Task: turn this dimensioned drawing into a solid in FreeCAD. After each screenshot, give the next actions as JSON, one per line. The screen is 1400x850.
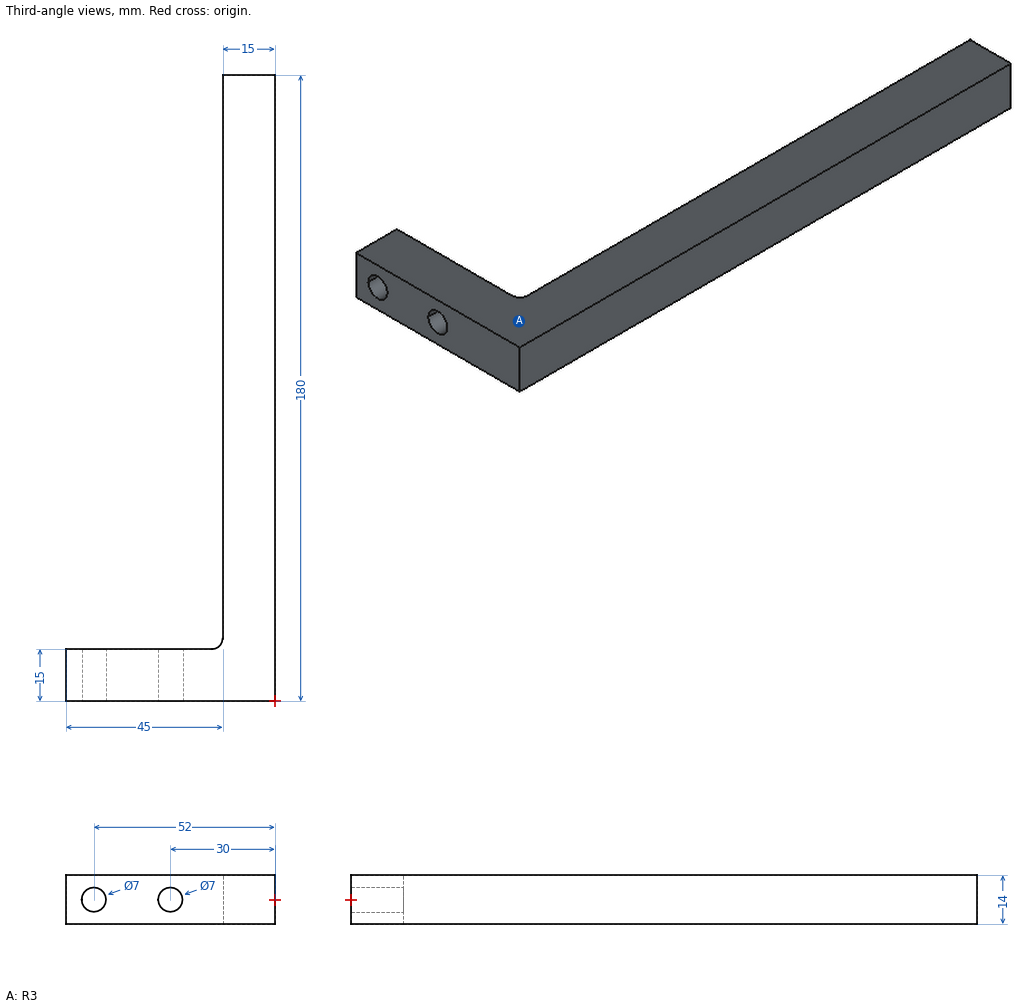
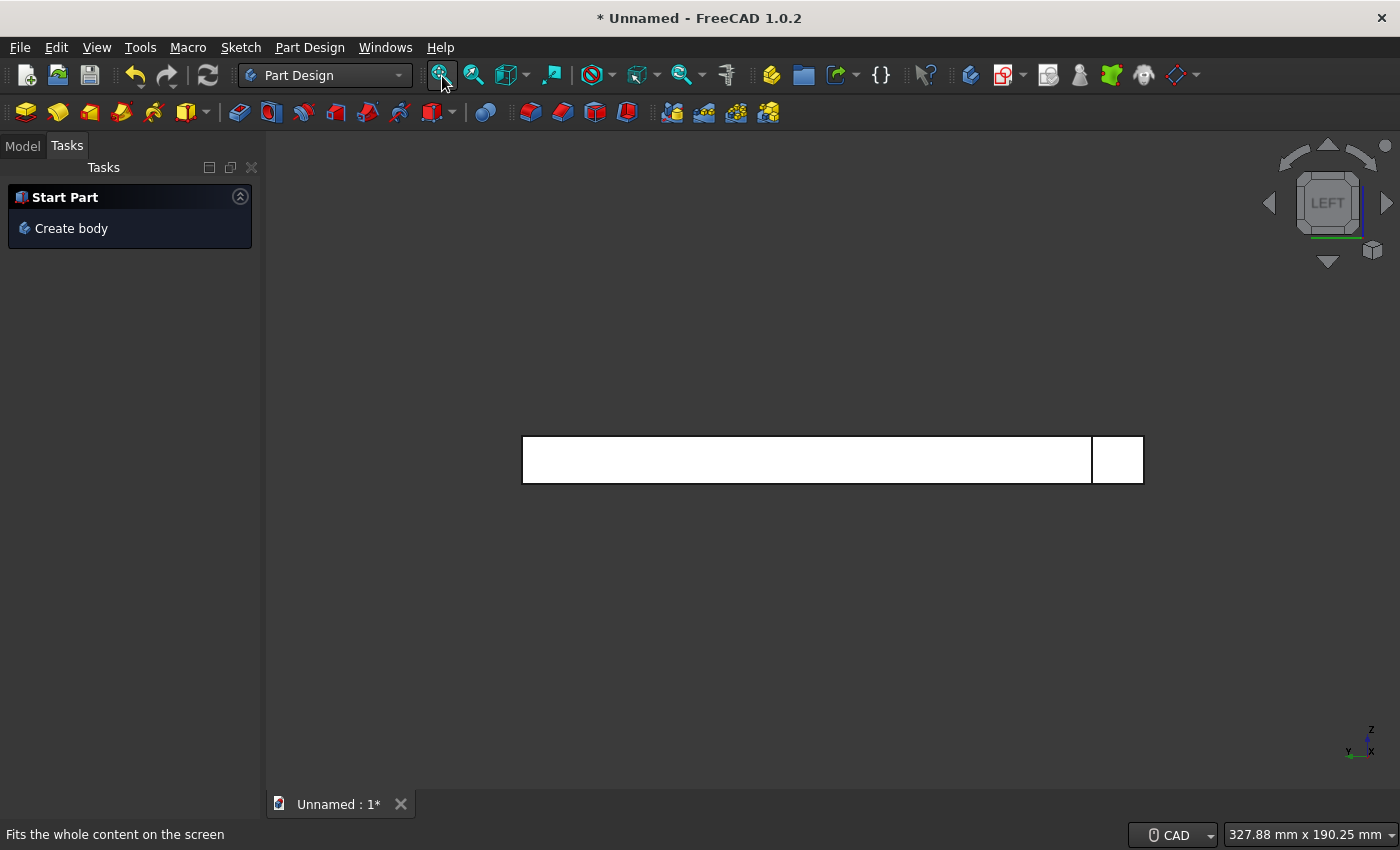
{"action": "key", "text": "v 3"}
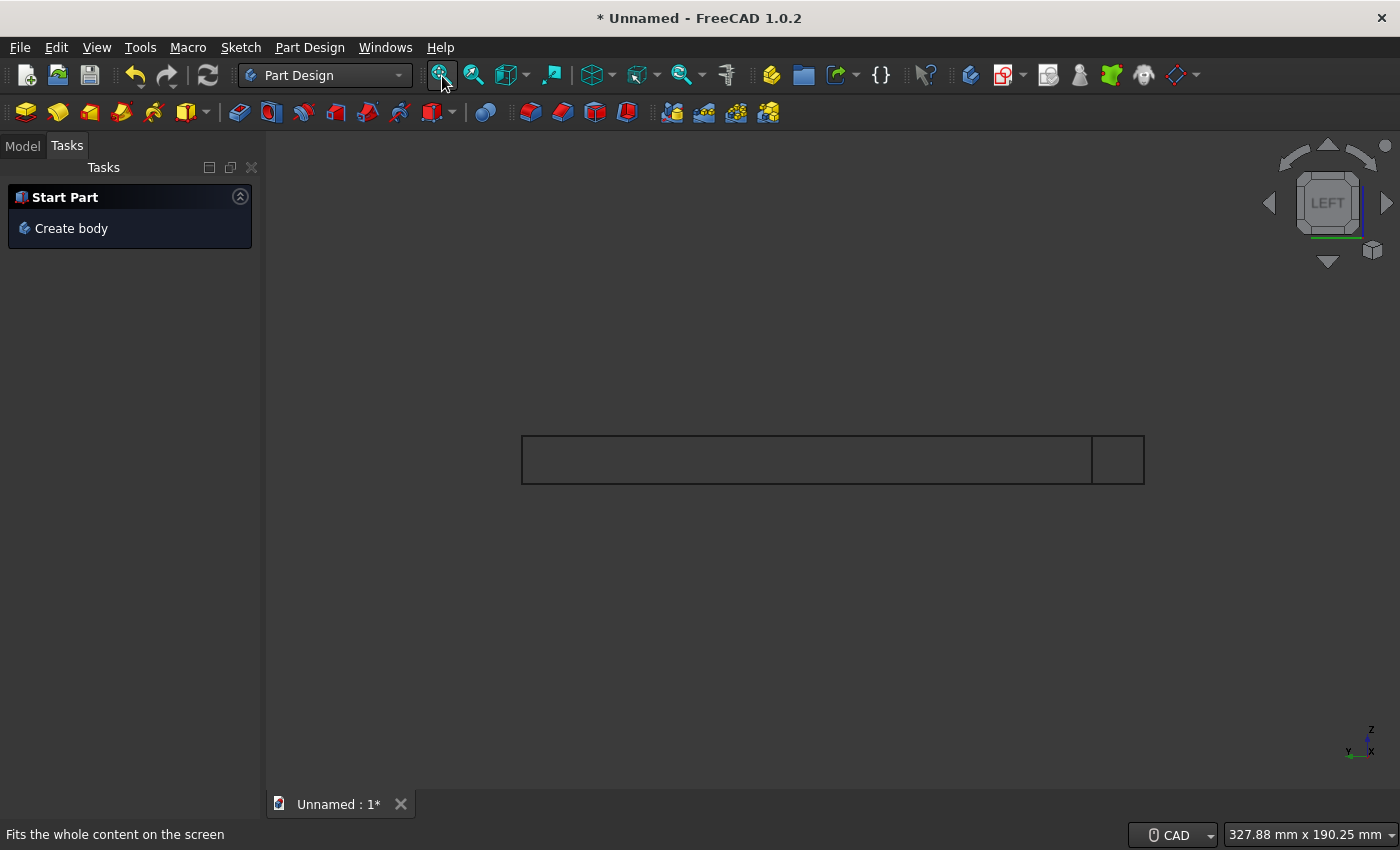
{"action": "key", "text": "0"}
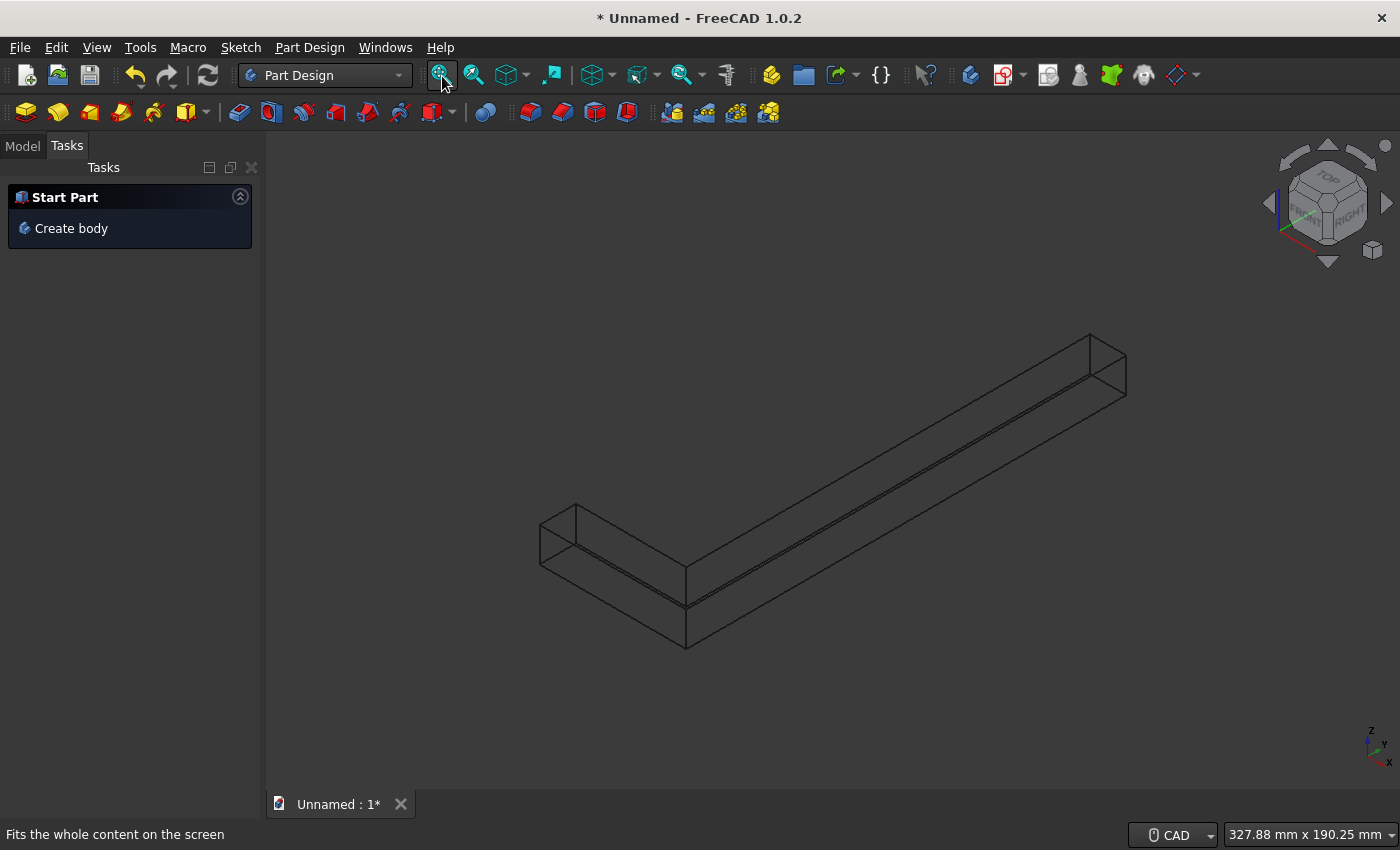
{"action": "left_click", "coordinate": [686, 586]}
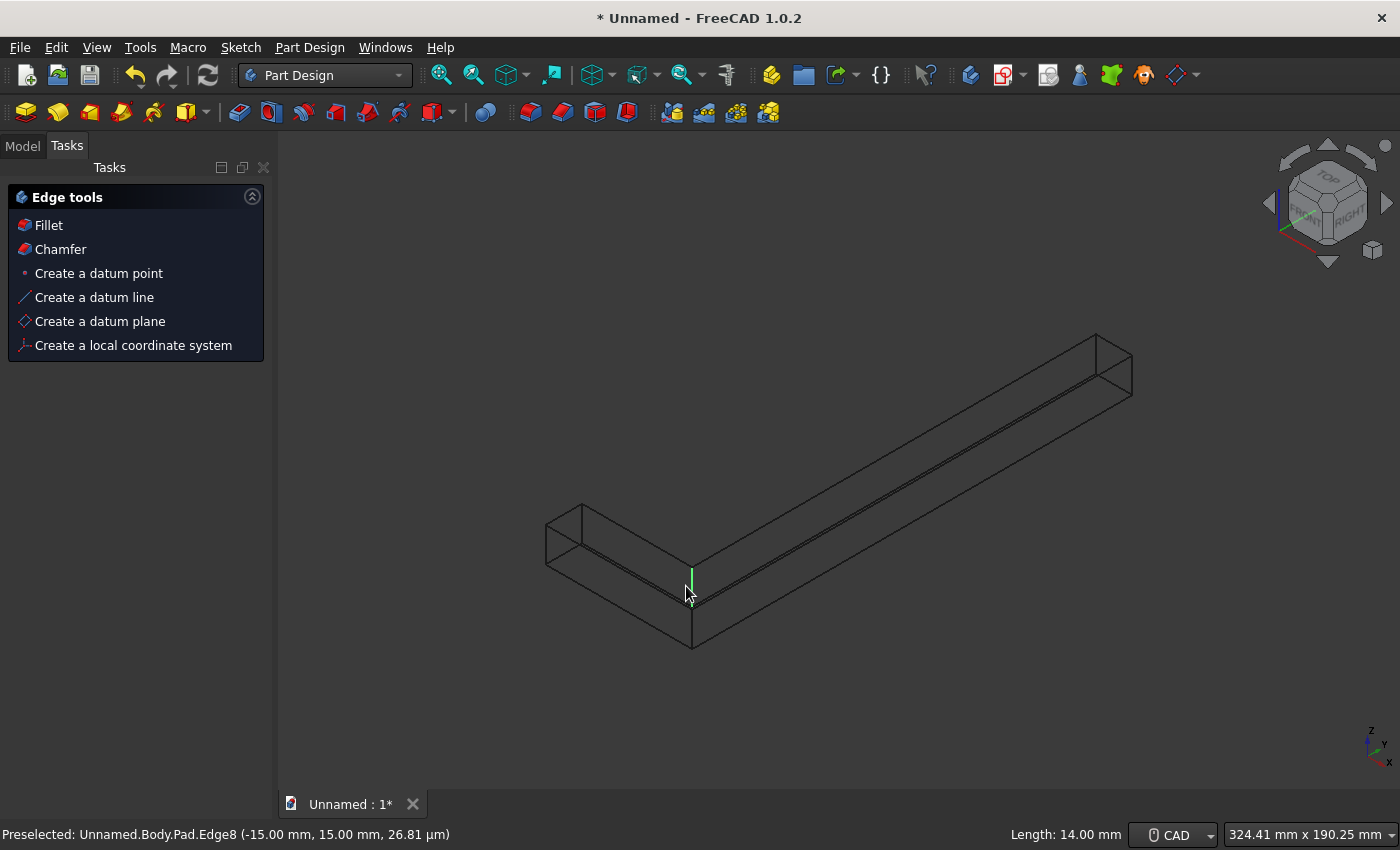
{"action": "key", "text": "v 1"}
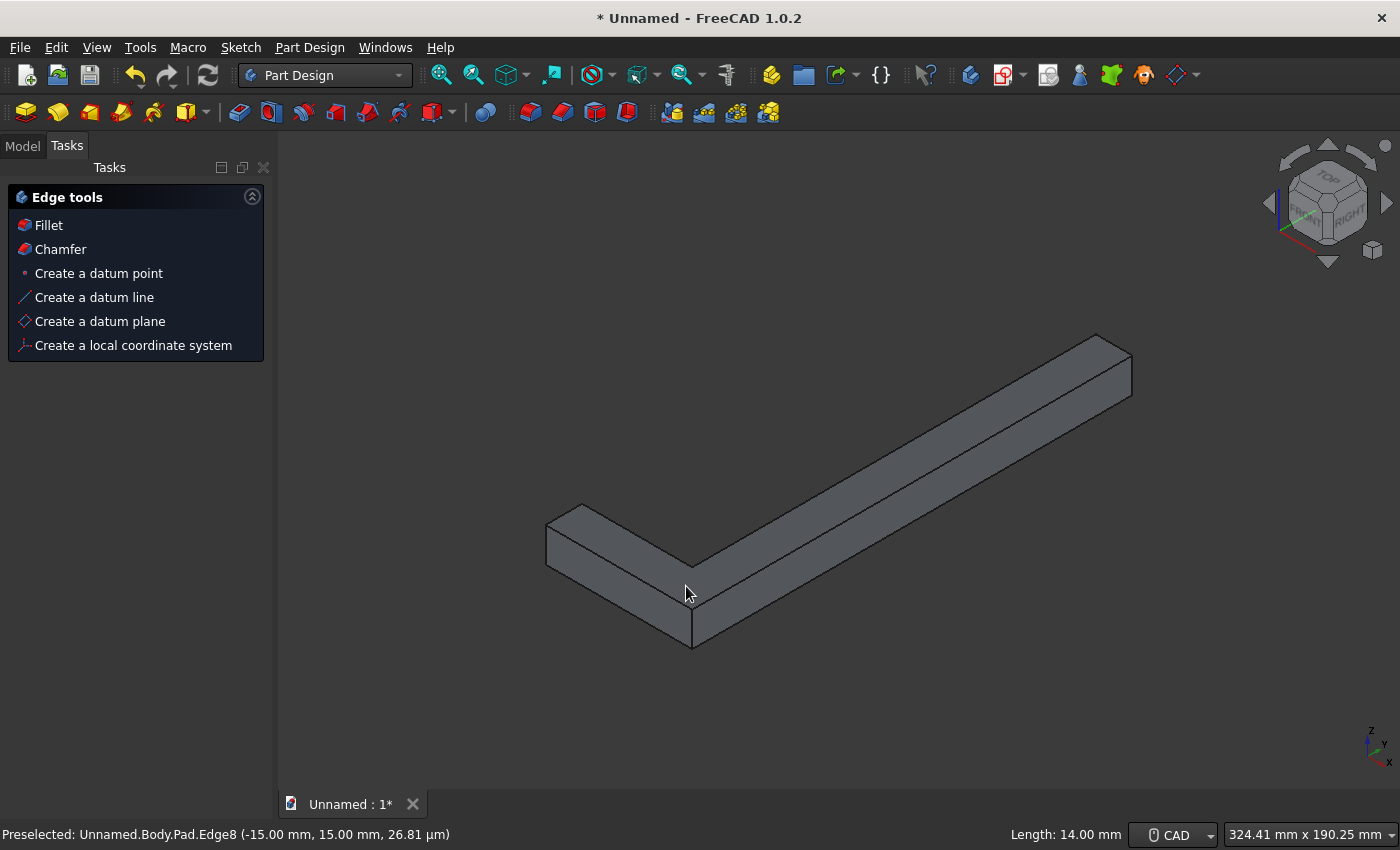
{"action": "left_click", "coordinate": [532, 112]}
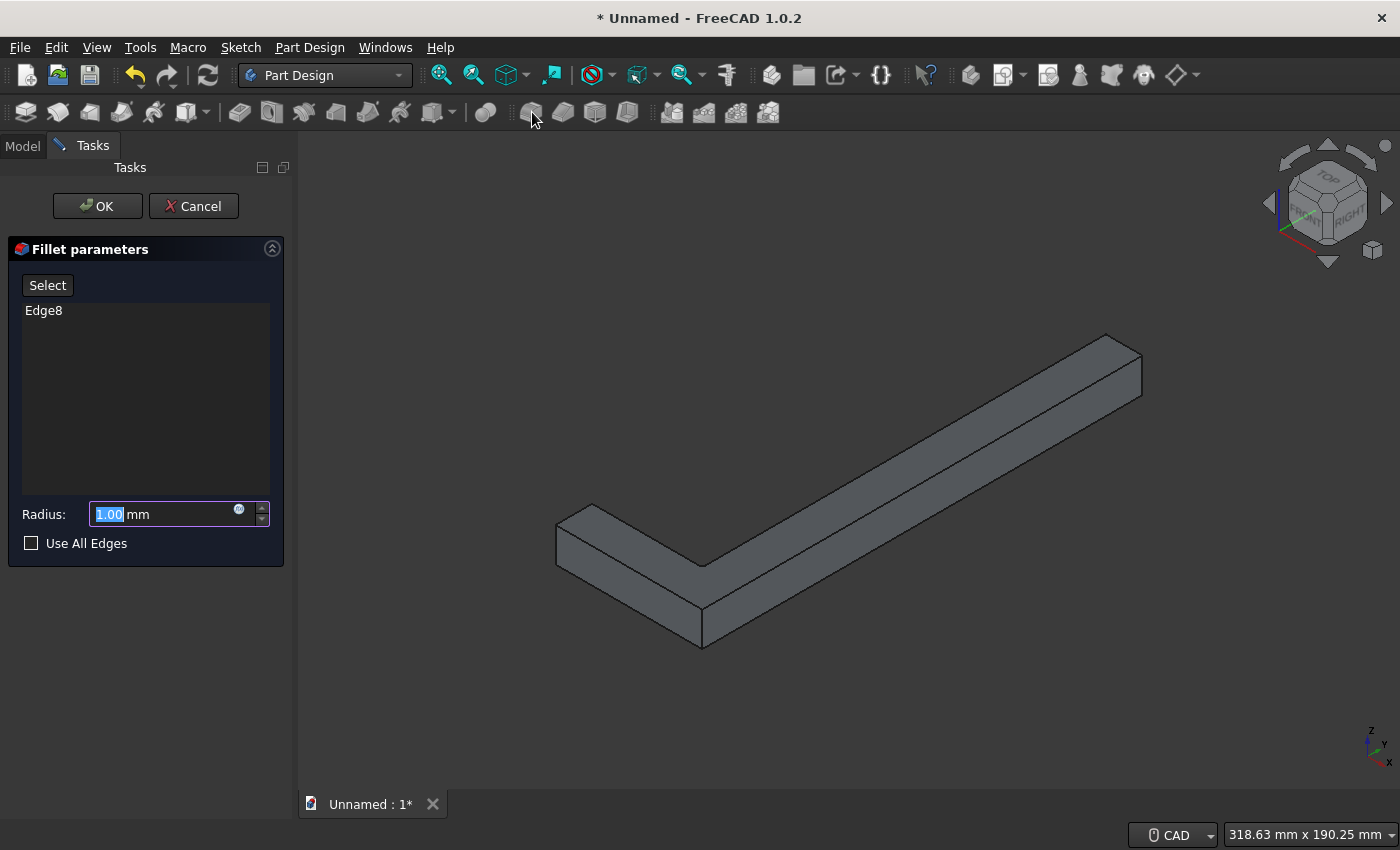
{"action": "type", "text": "3"}
{"action": "key", "text": "Tab"}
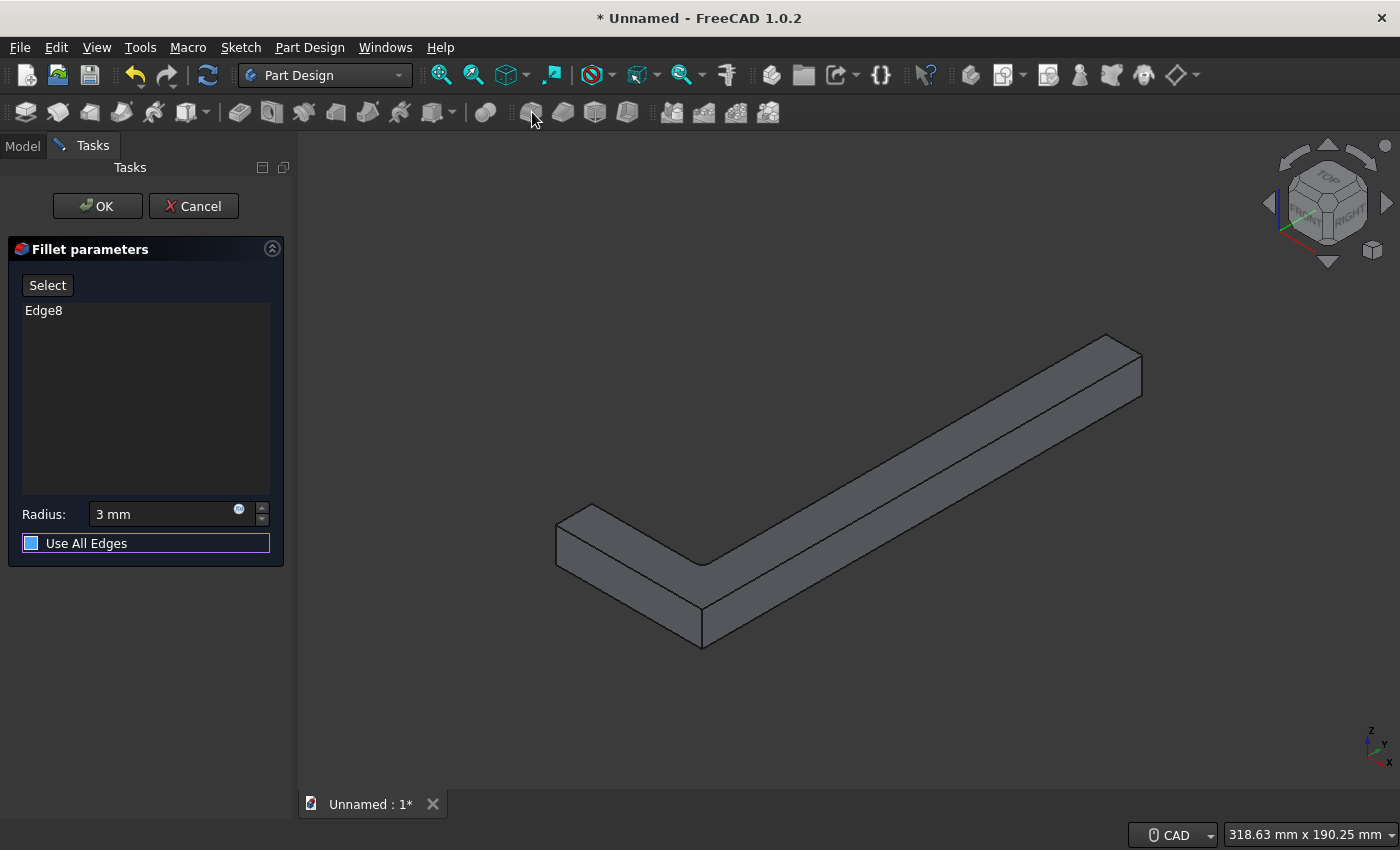
{"action": "left_click", "coordinate": [98, 206]}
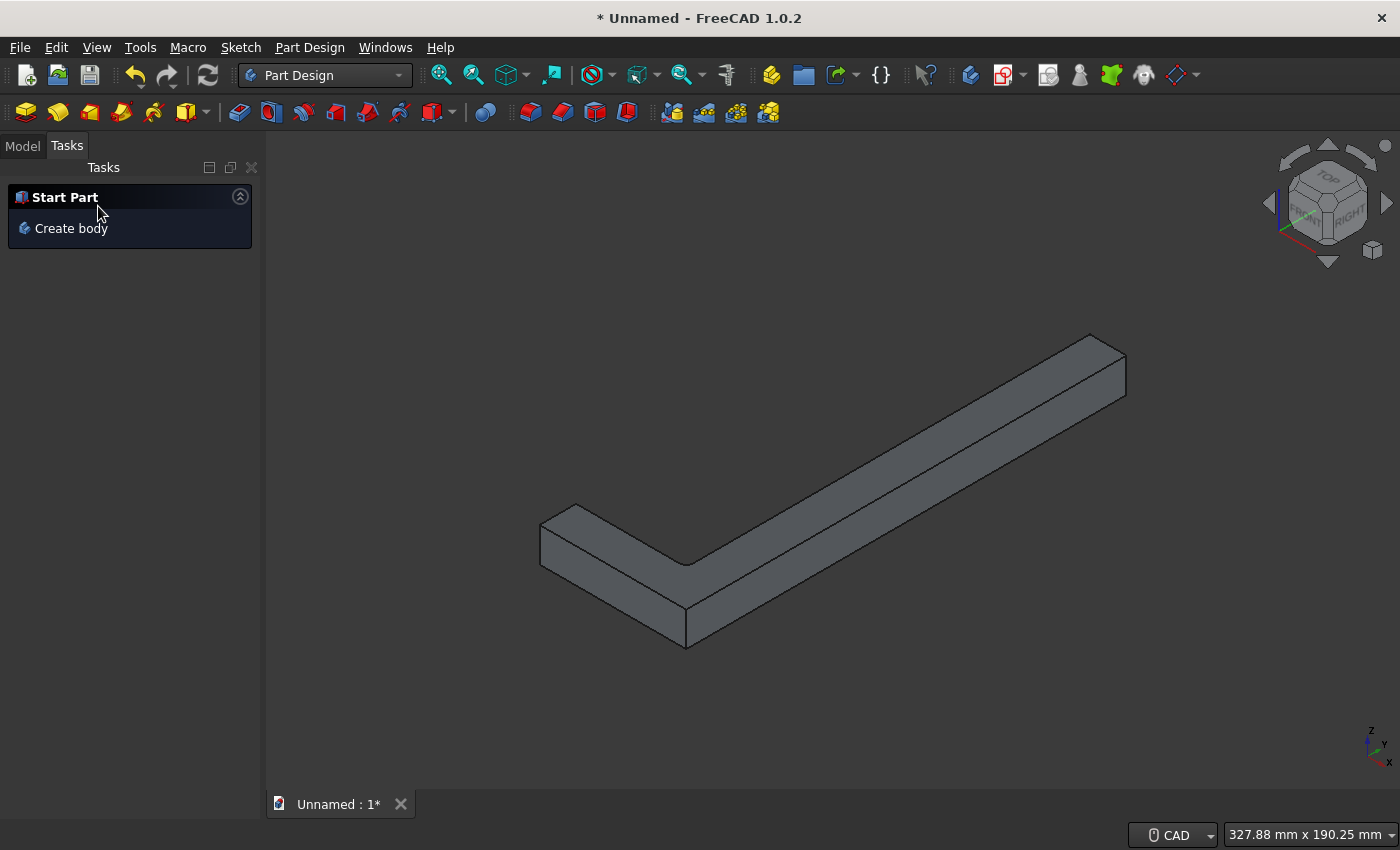
{"action": "key", "text": "4"}